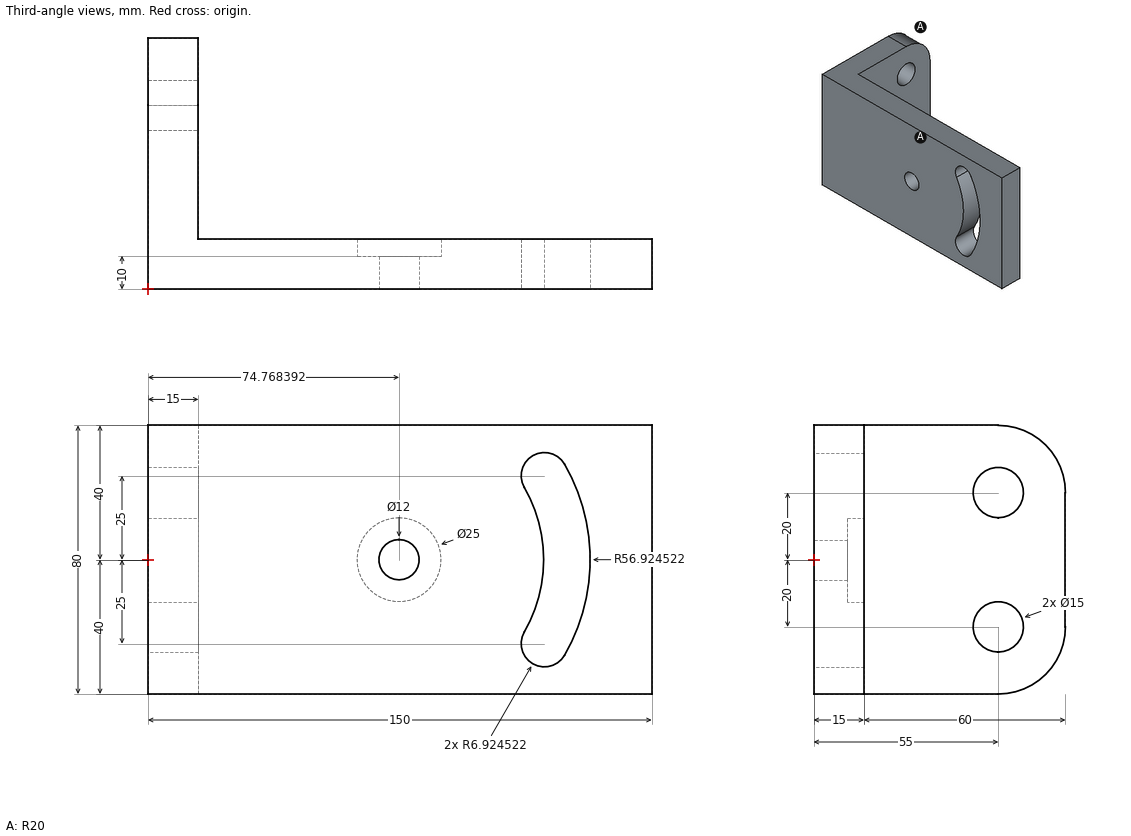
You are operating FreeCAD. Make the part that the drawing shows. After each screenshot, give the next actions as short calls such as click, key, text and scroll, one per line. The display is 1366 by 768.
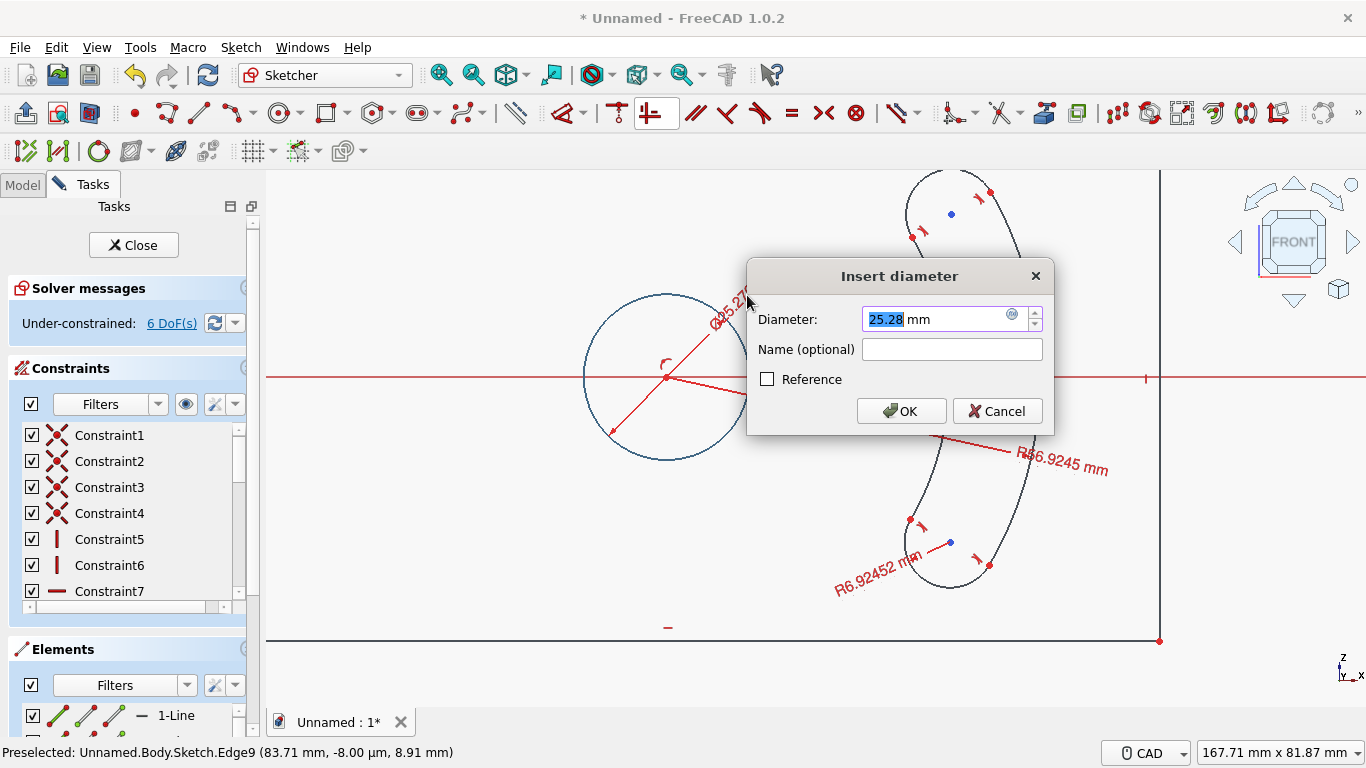
text(25)
key(Return)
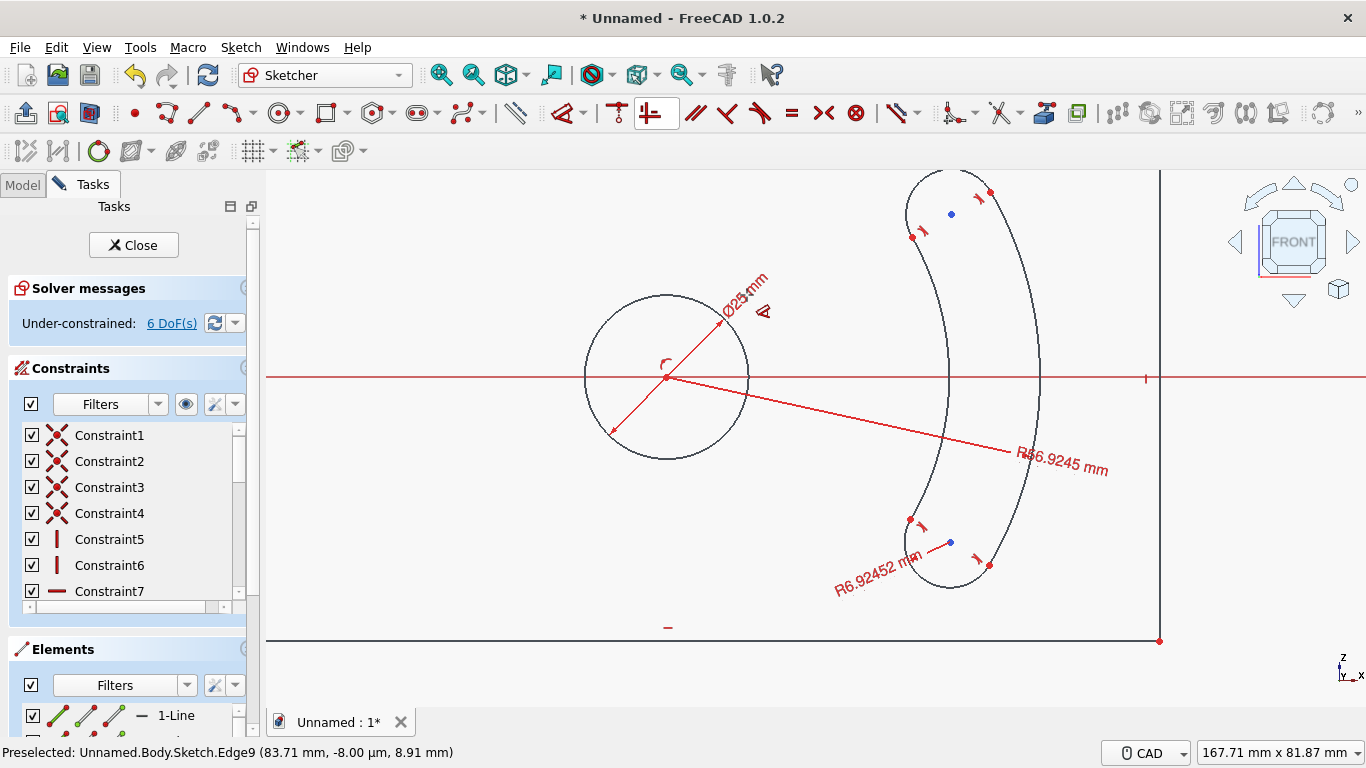
scroll(909, 563, down, 2)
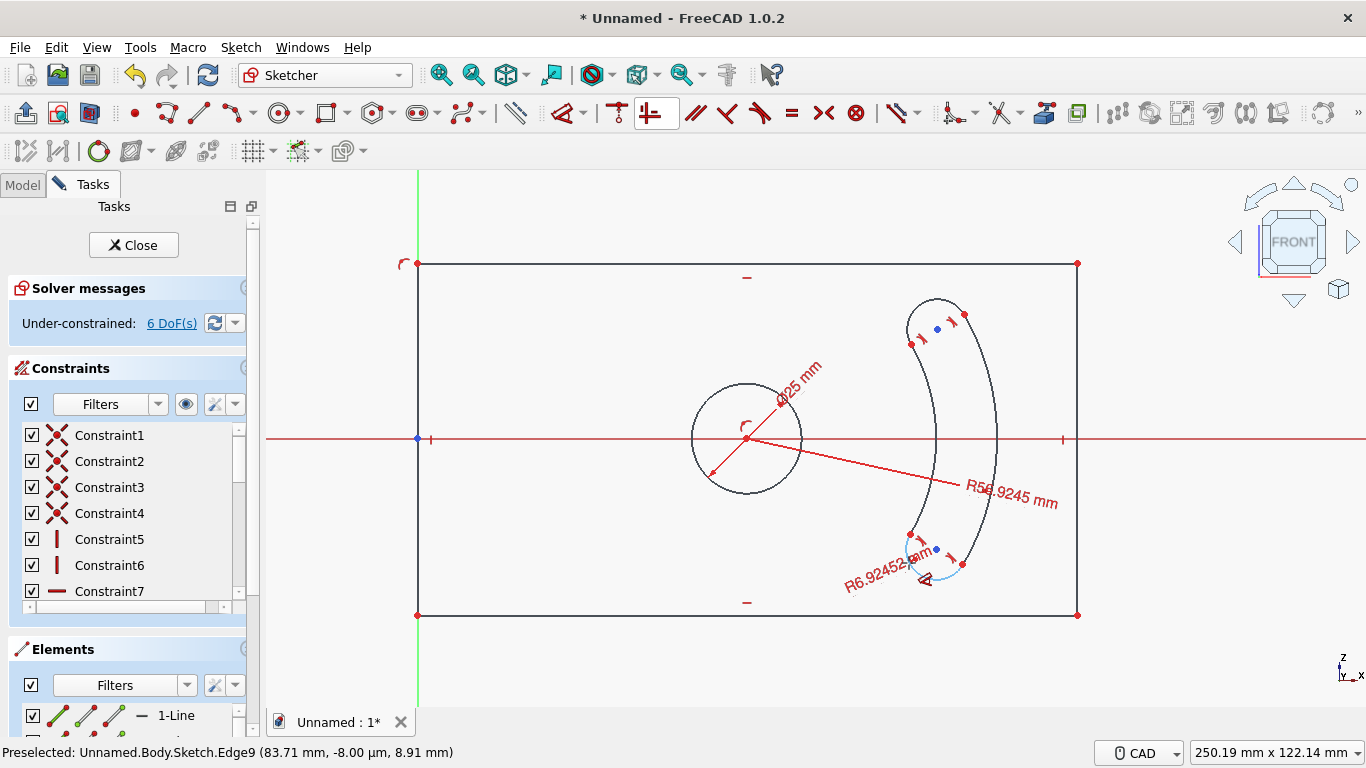
click(418, 369)
click(384, 359)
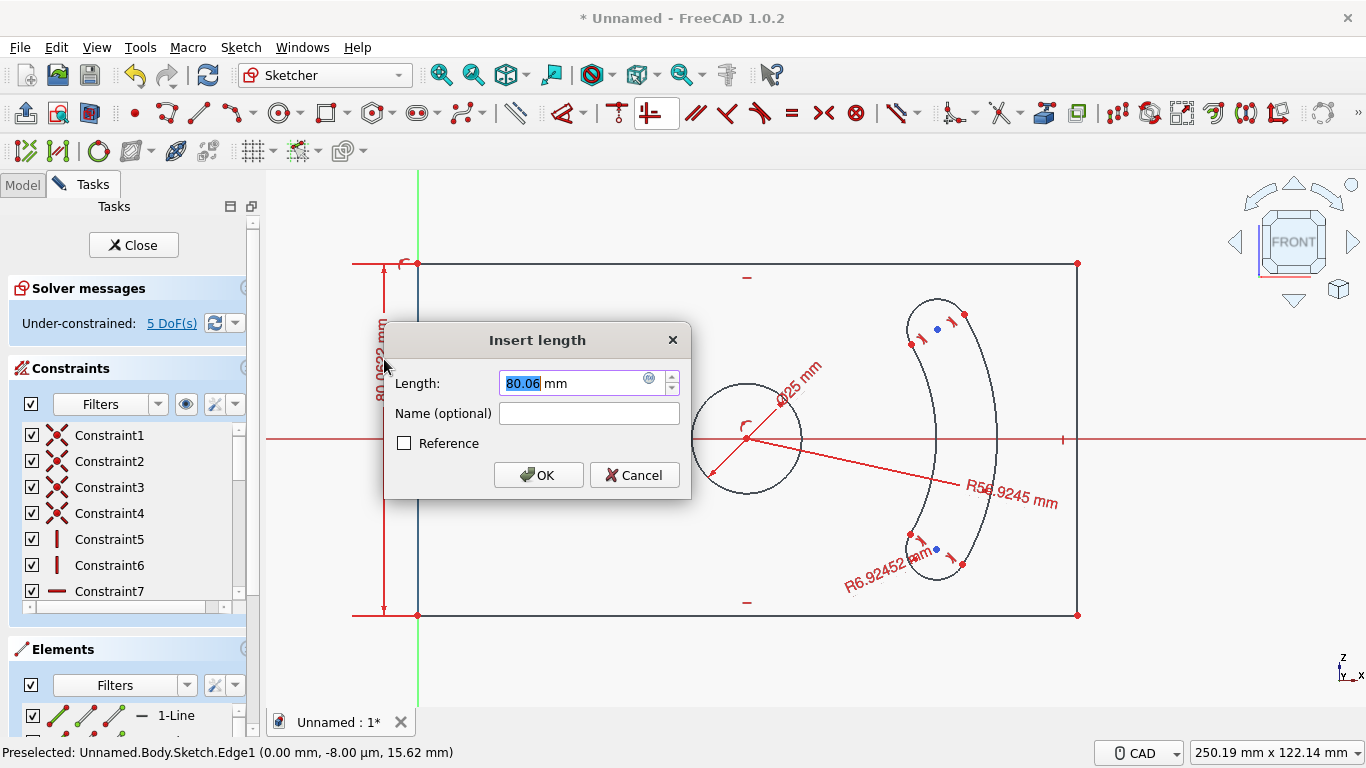
text(80)
key(Return)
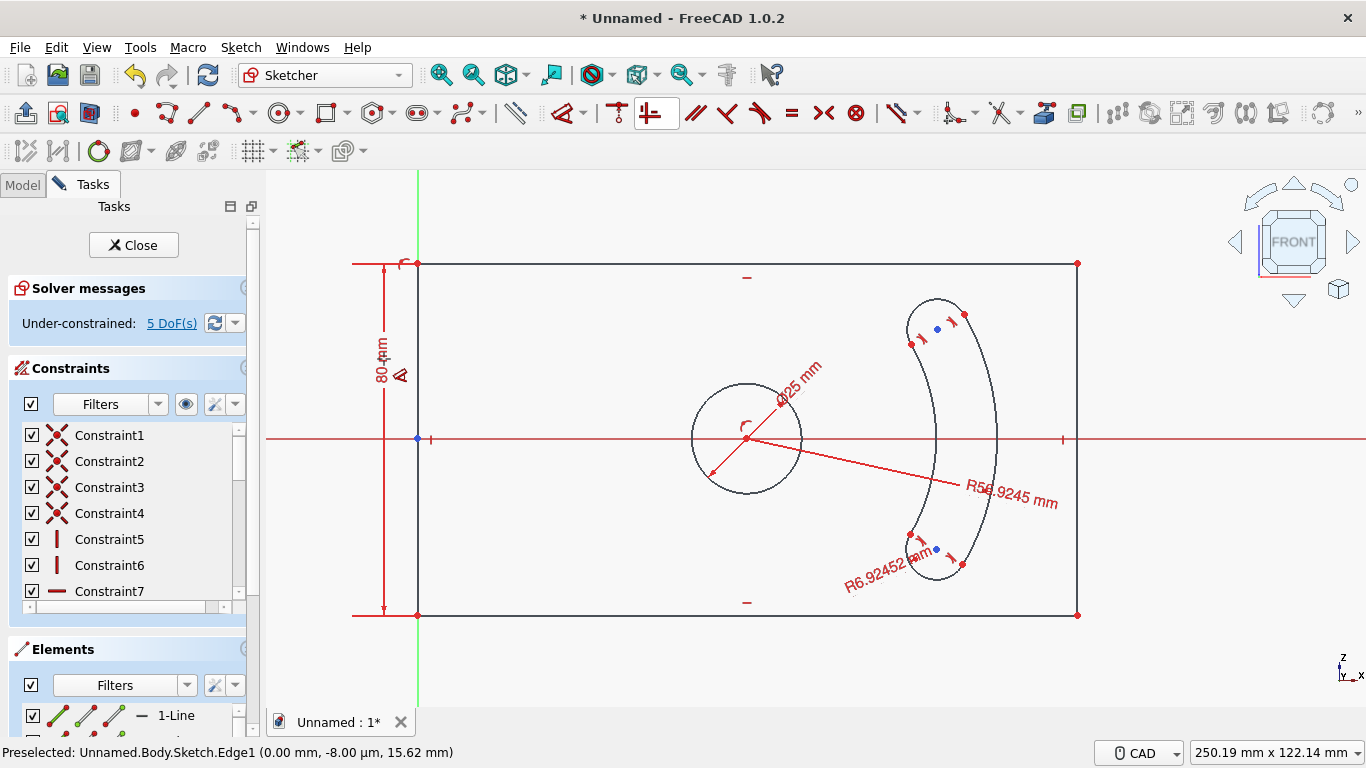
click(616, 616)
click(748, 650)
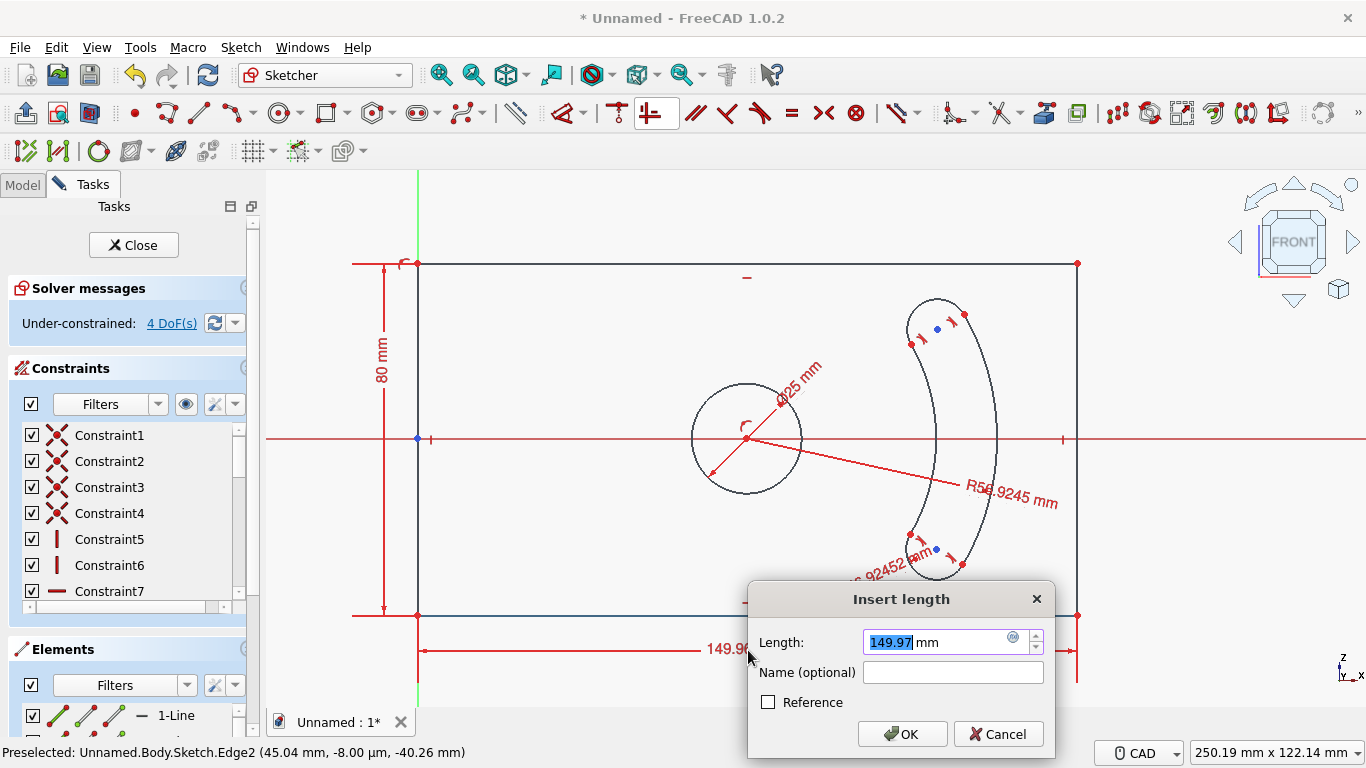
text(150)
key(Return)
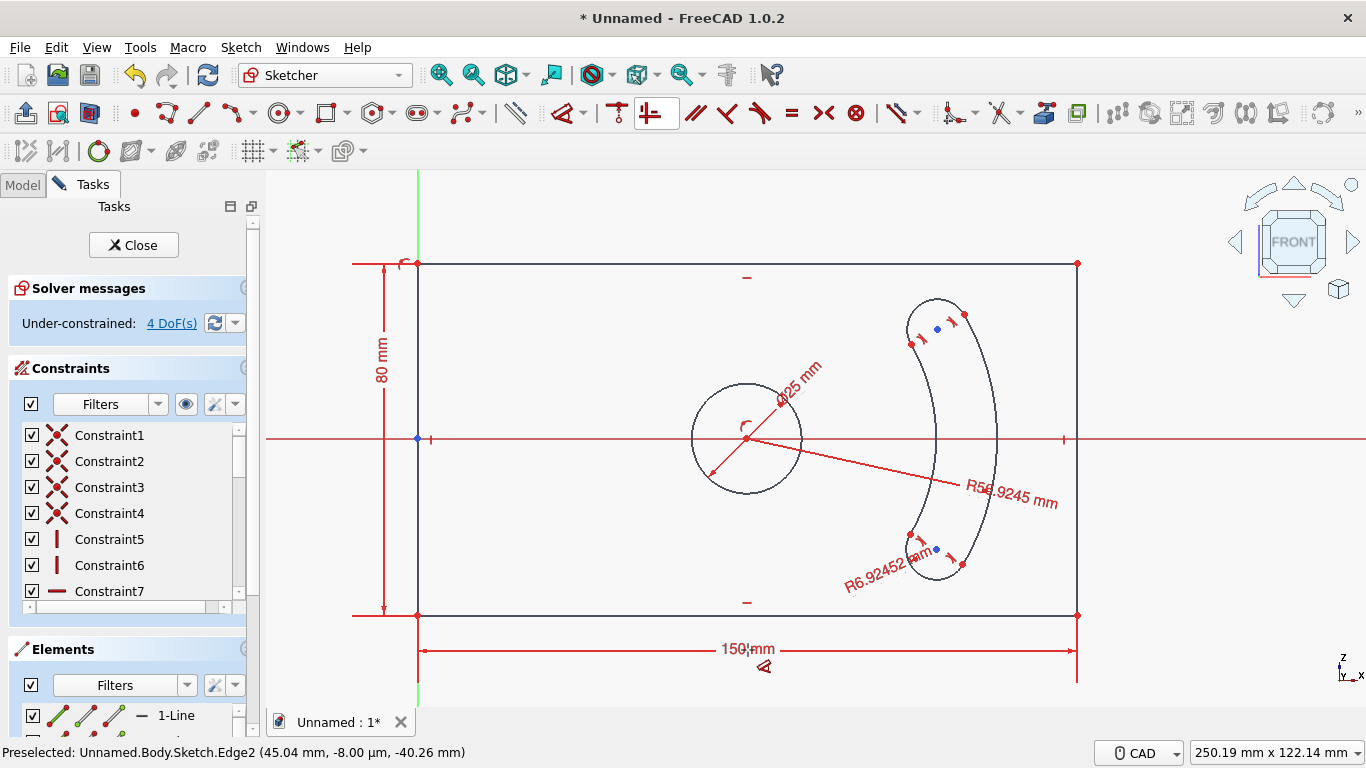
click(418, 264)
click(384, 311)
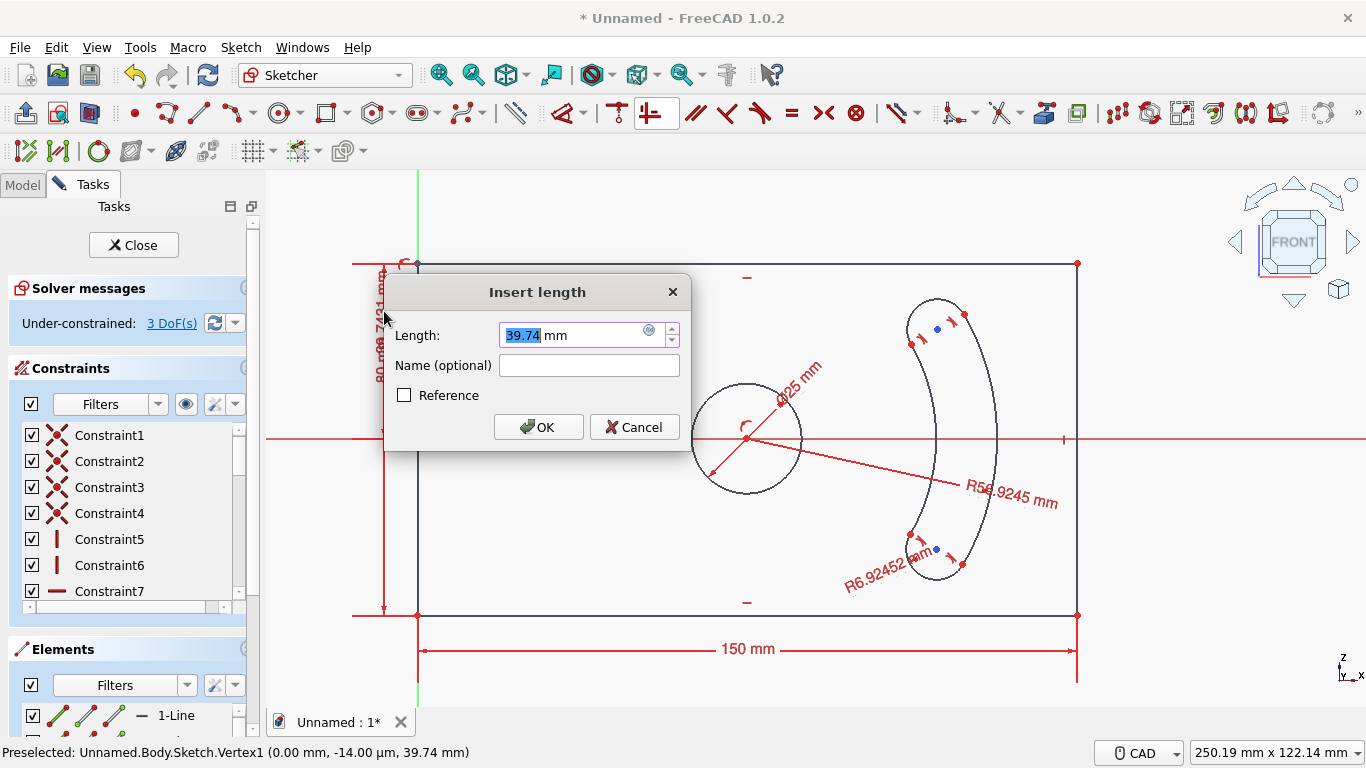
text(40)
key(Return)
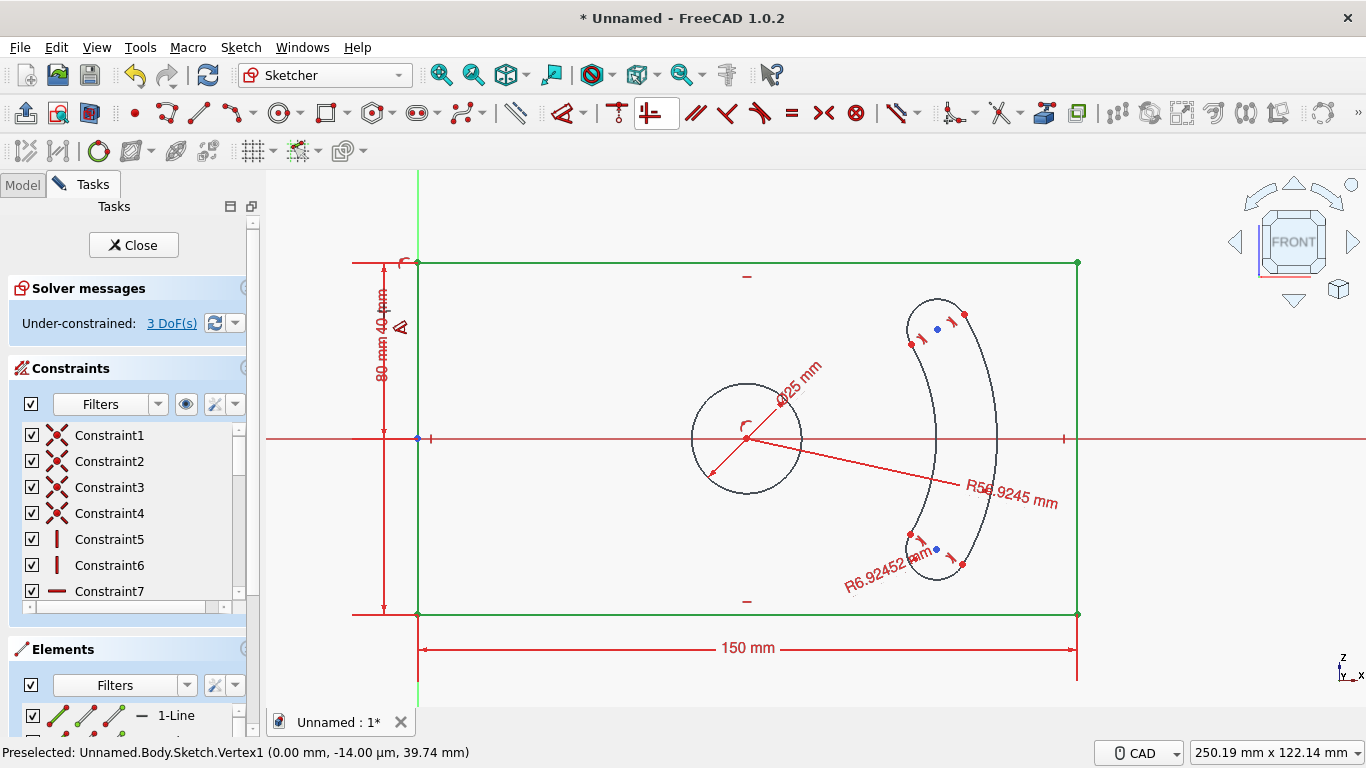
click(937, 549)
click(384, 494)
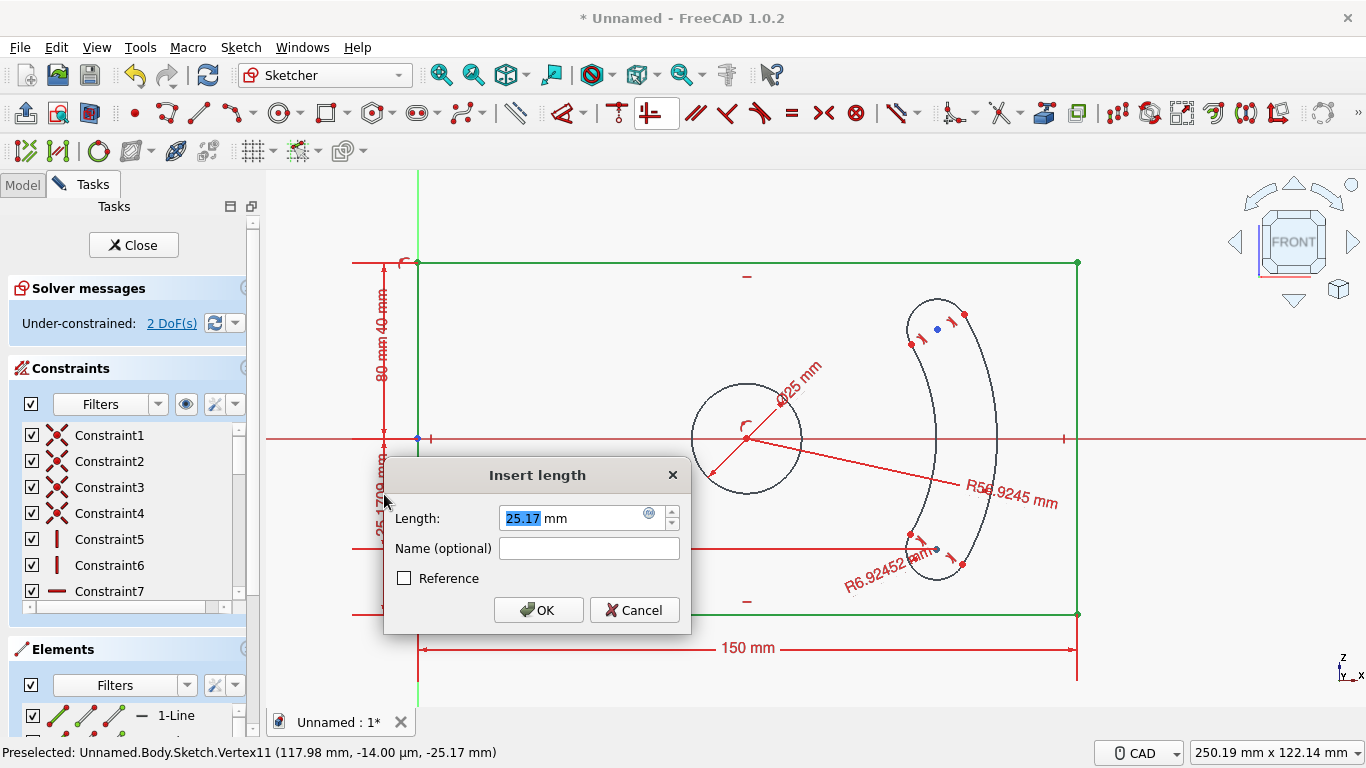
text(25)
key(Return)